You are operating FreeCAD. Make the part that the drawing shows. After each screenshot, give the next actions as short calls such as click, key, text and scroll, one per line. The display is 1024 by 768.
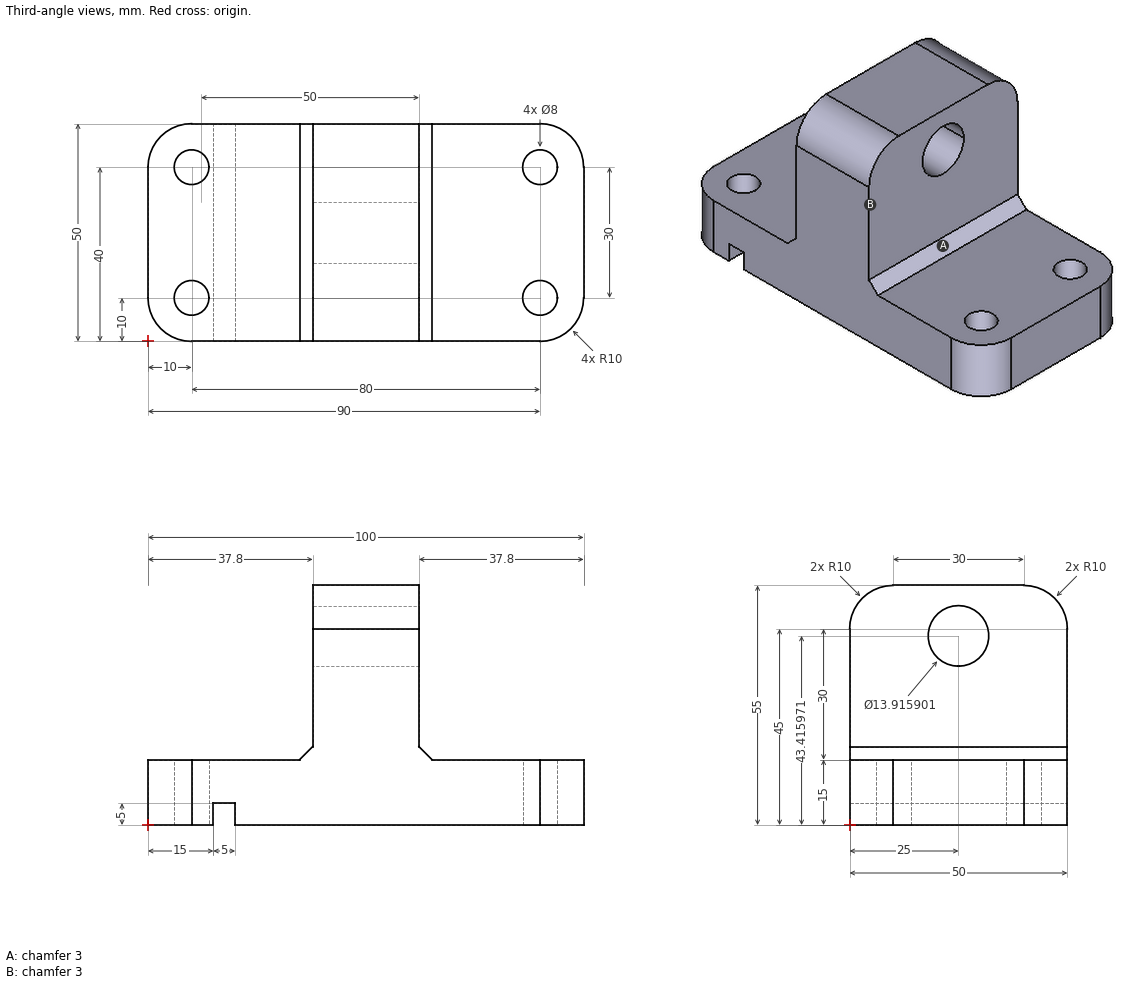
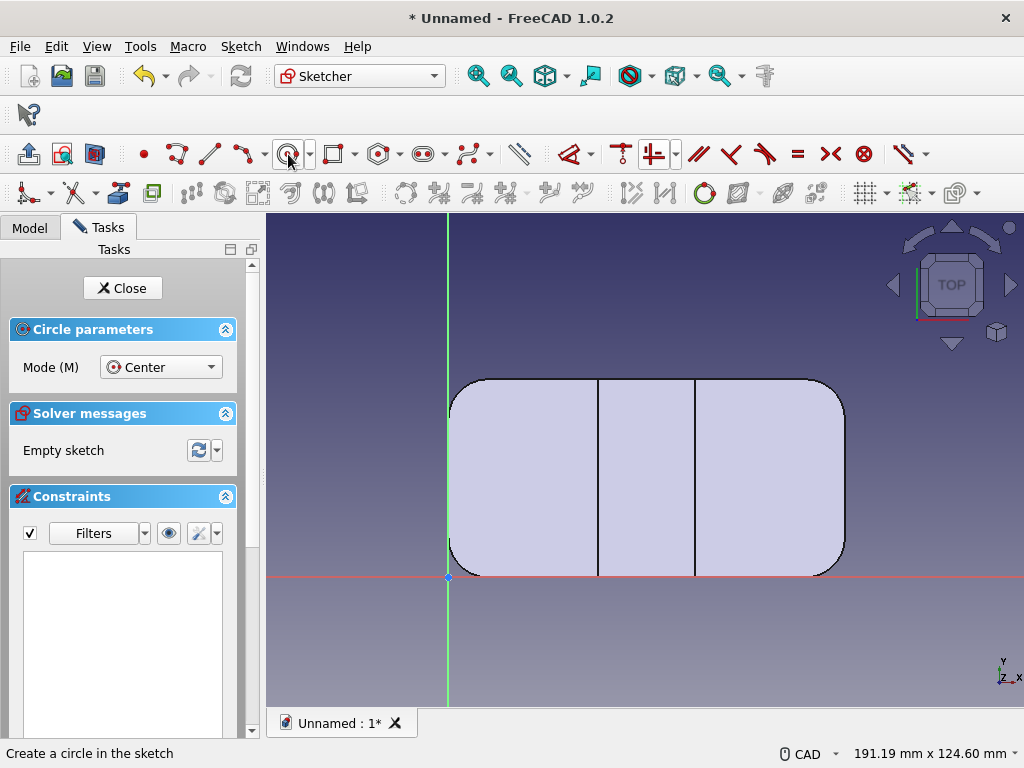
scroll(805, 419, up, 2)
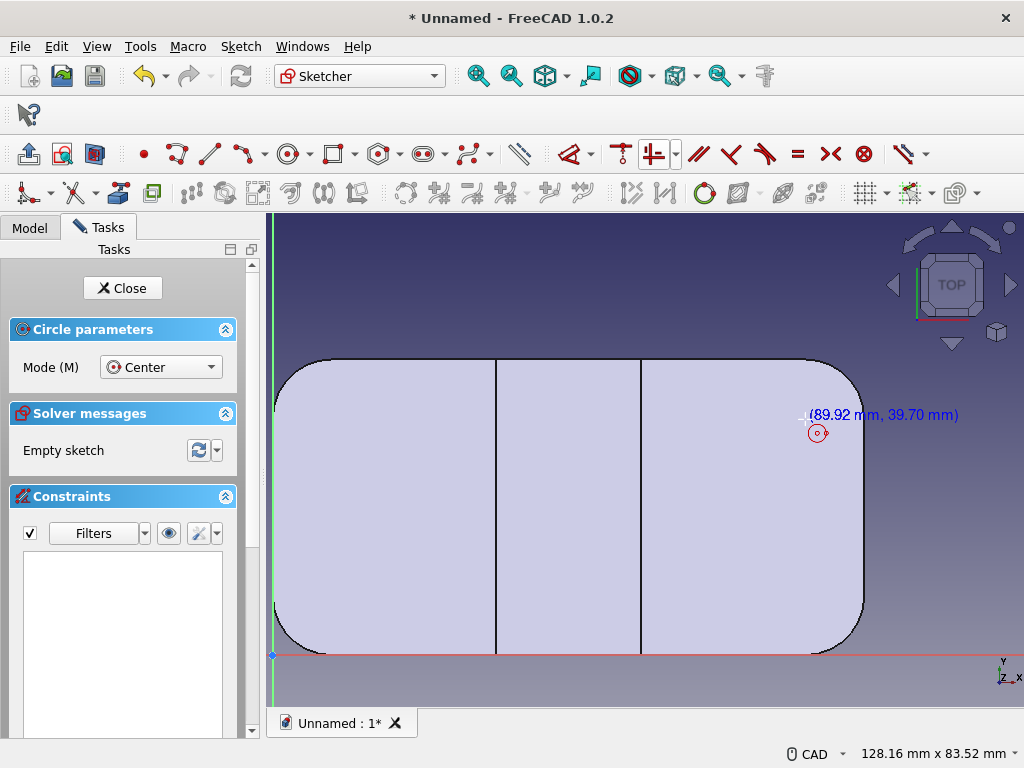
click(805, 419)
click(822, 402)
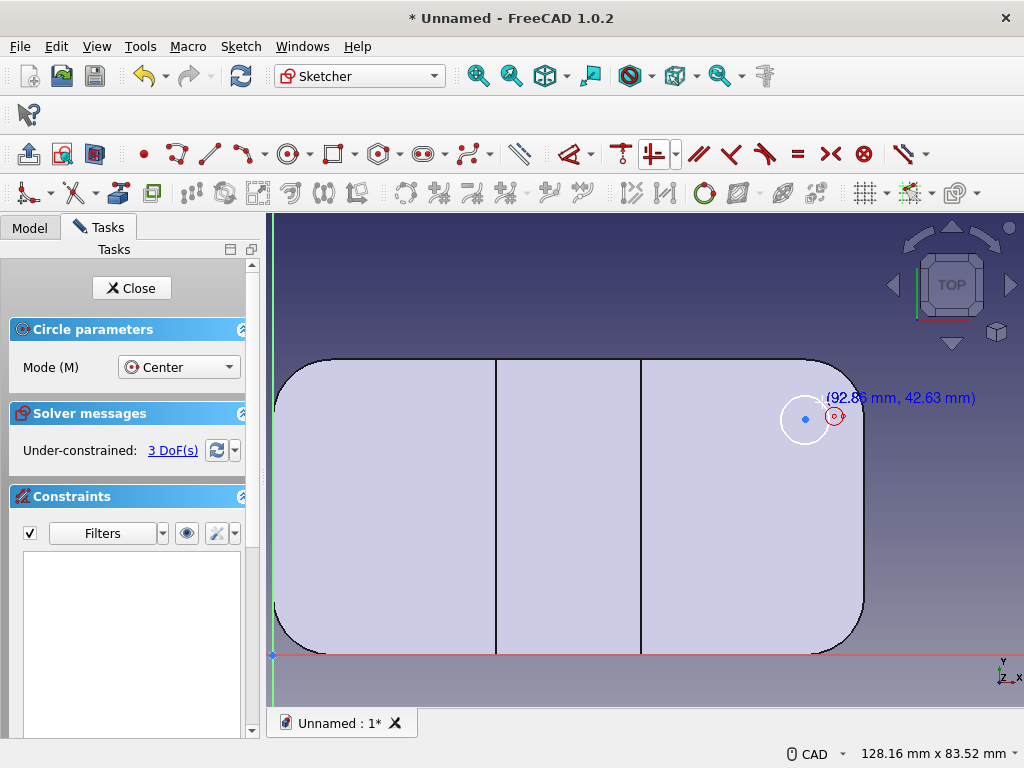
click(805, 596)
click(822, 579)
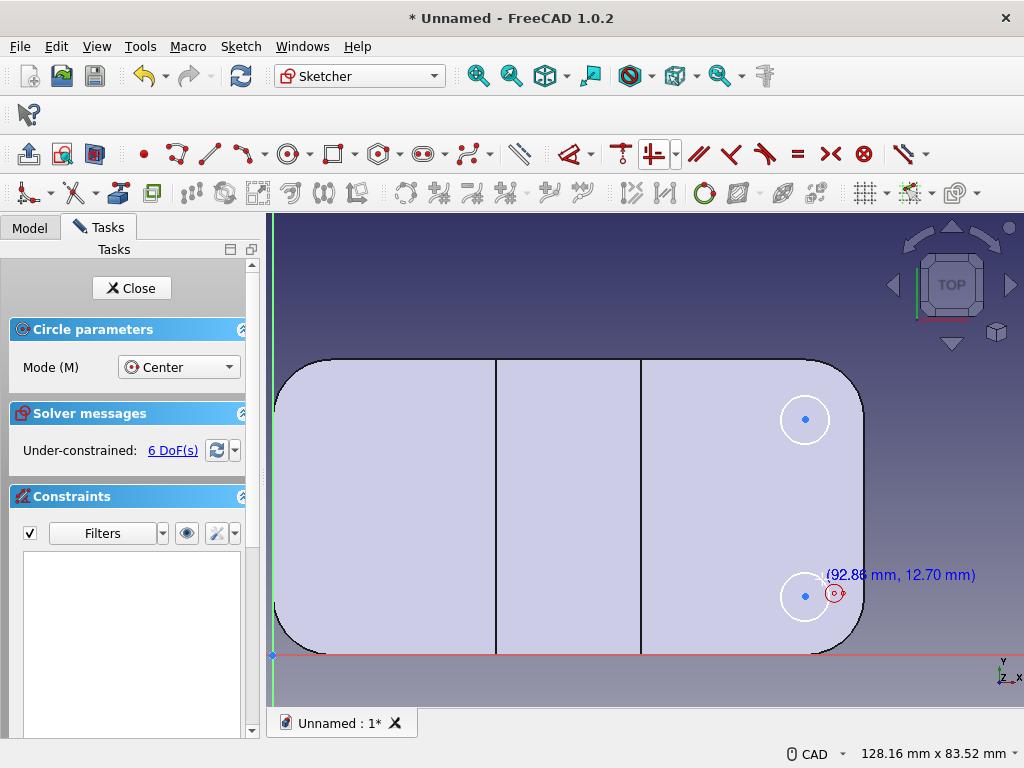
click(332, 419)
click(349, 402)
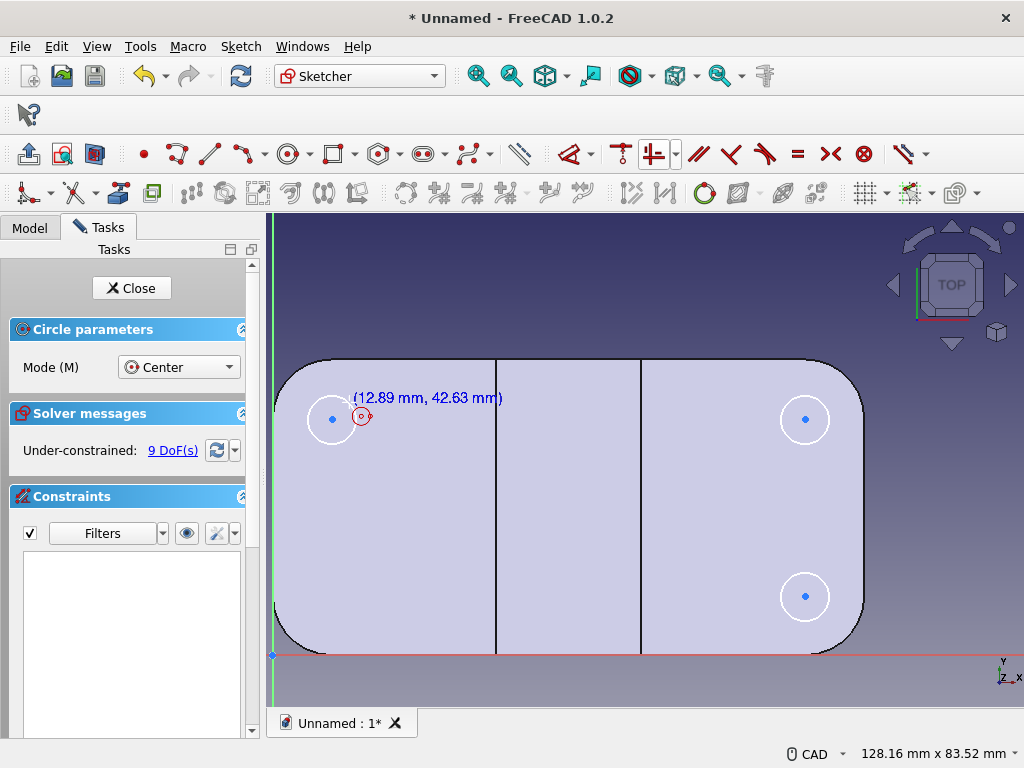
click(332, 596)
click(349, 579)
key(Escape)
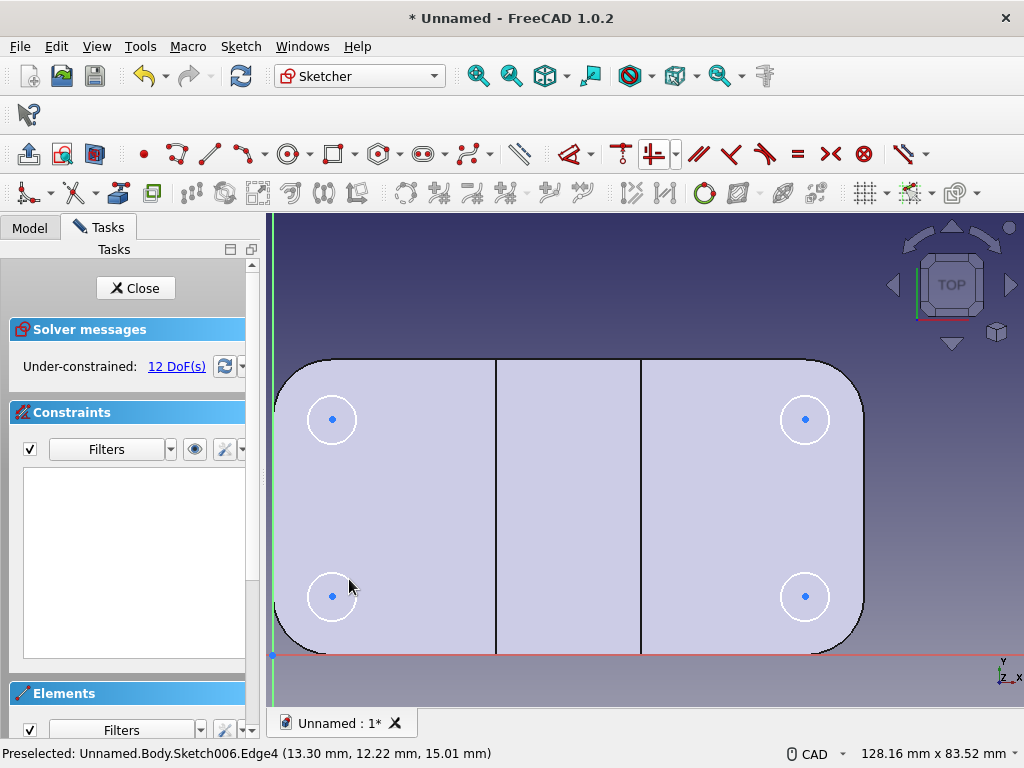
click(822, 403)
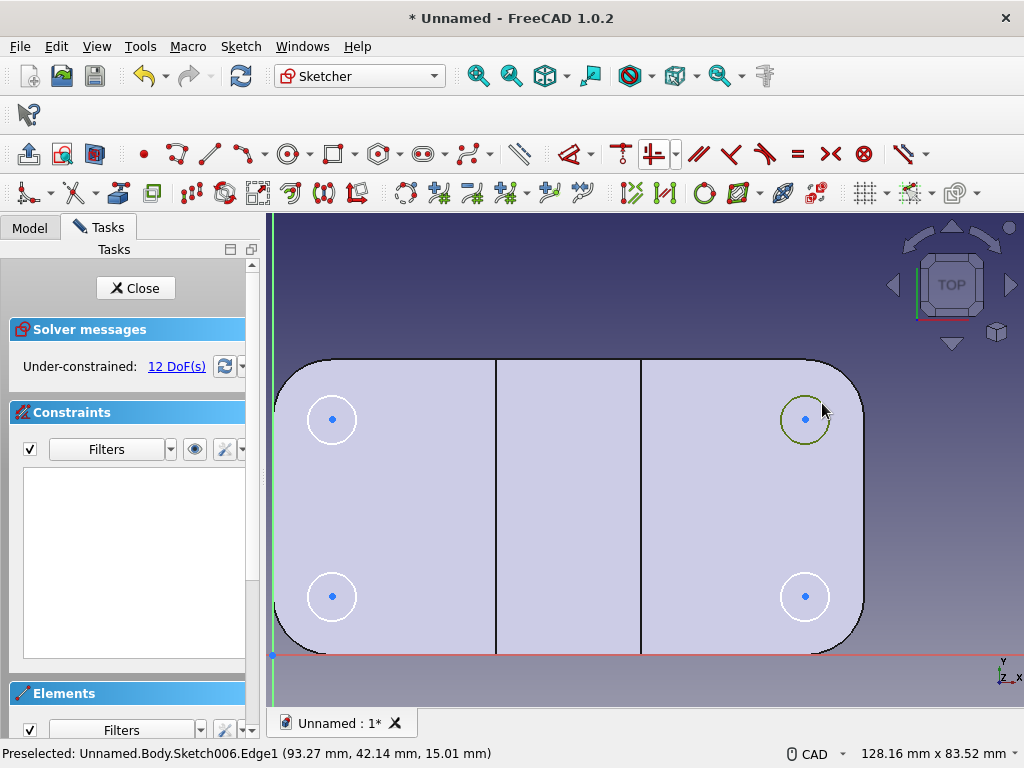
click(822, 580)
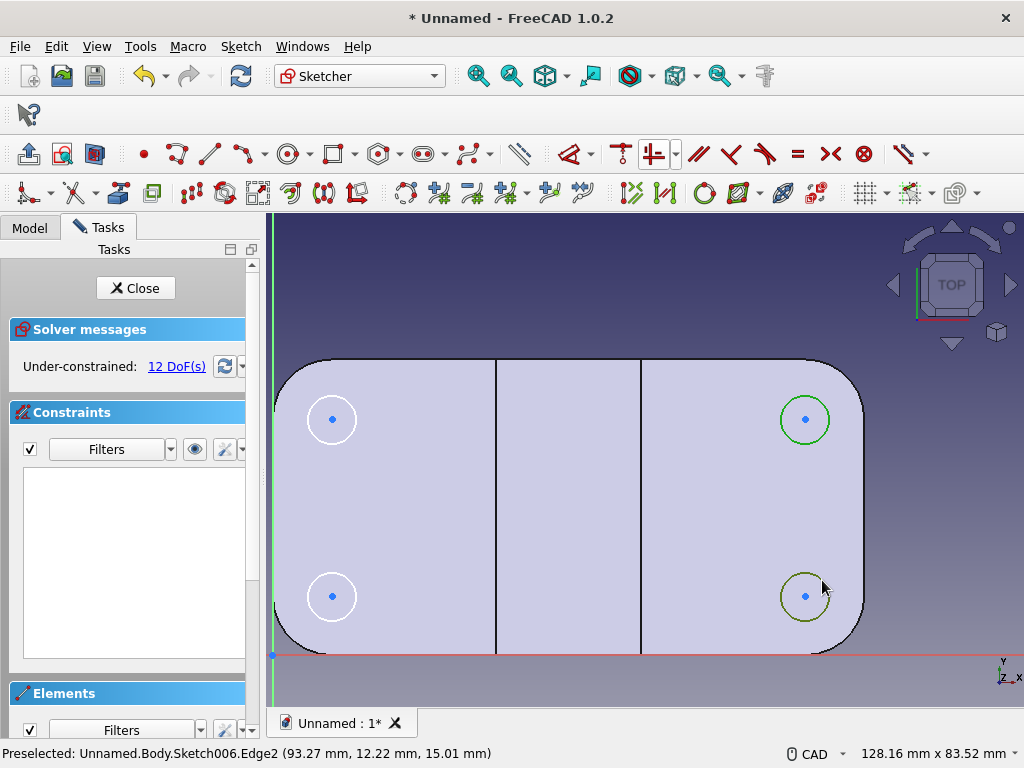
click(349, 403)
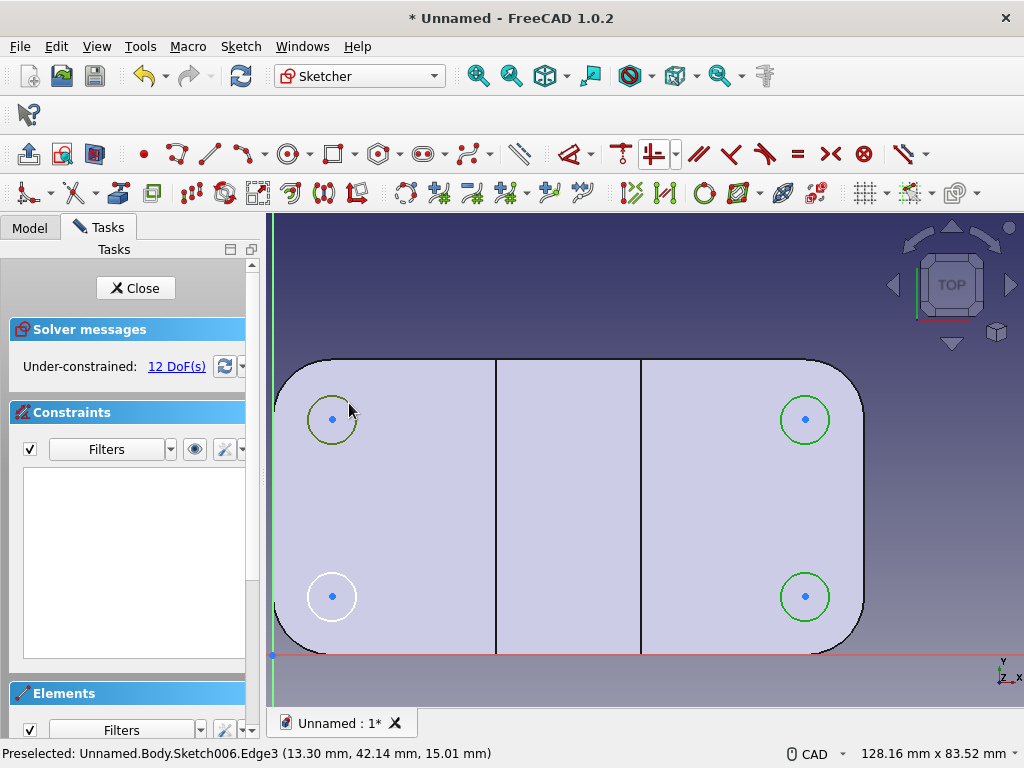
click(349, 580)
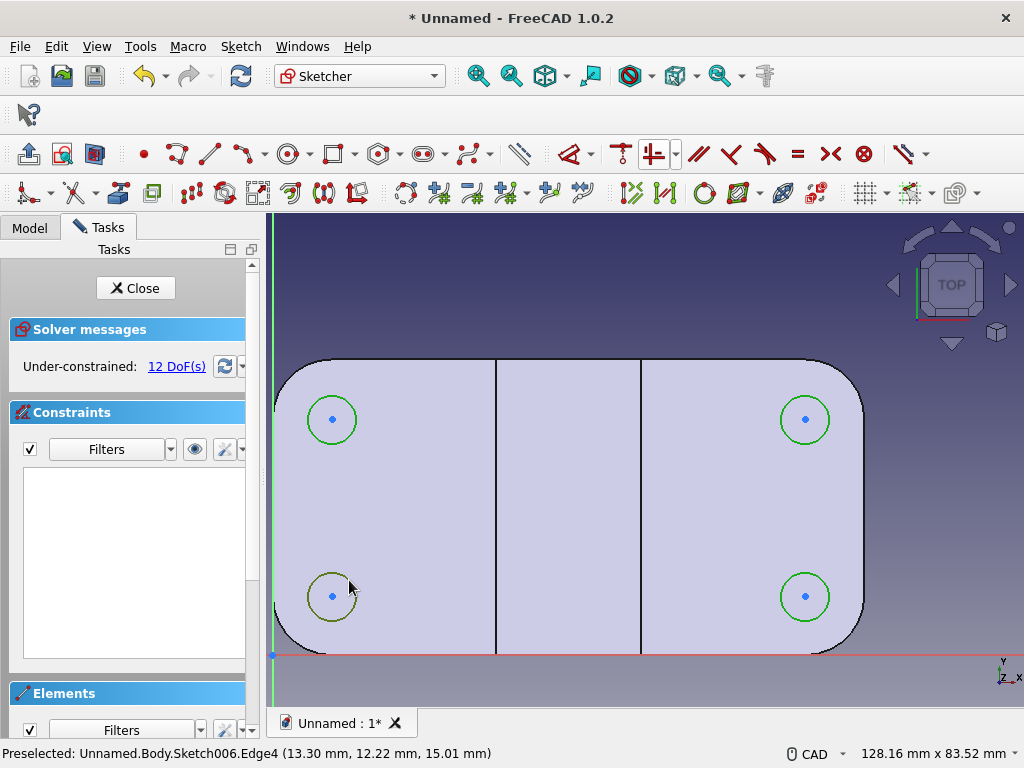
click(798, 154)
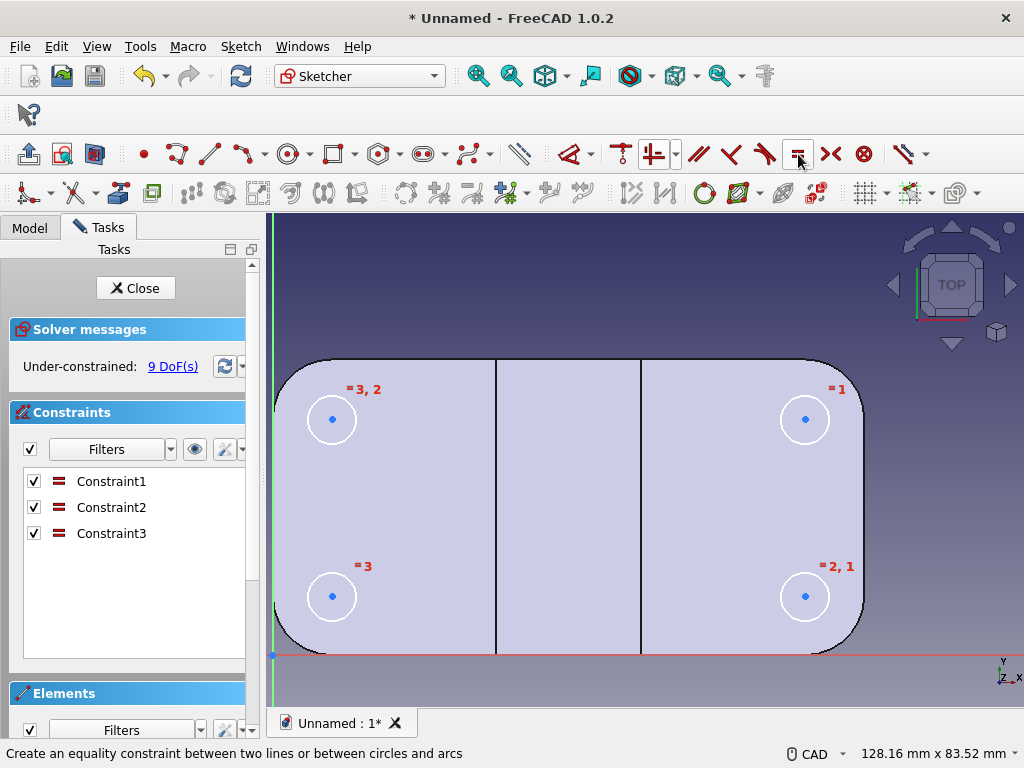
click(805, 420)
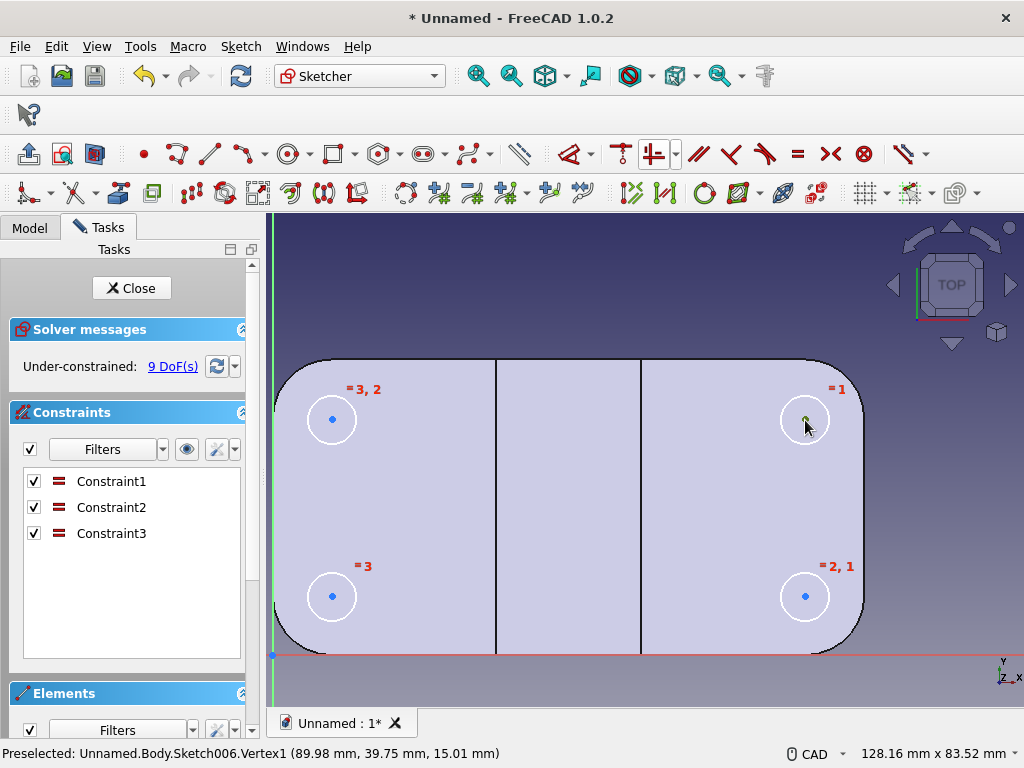
click(805, 597)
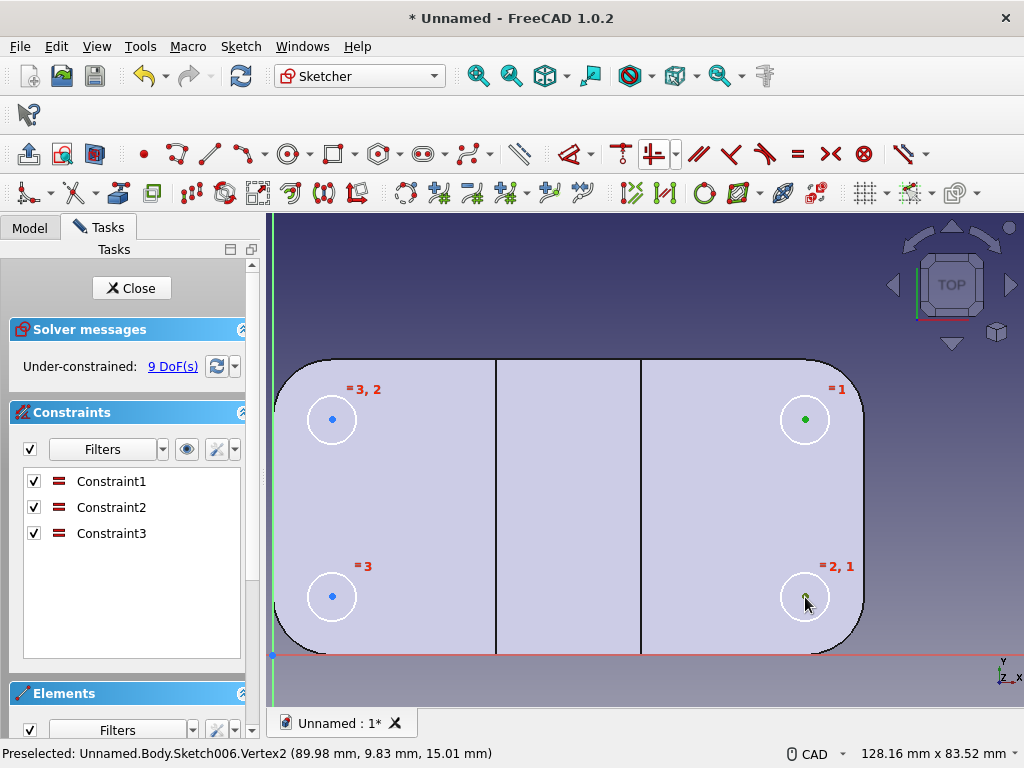
click(676, 154)